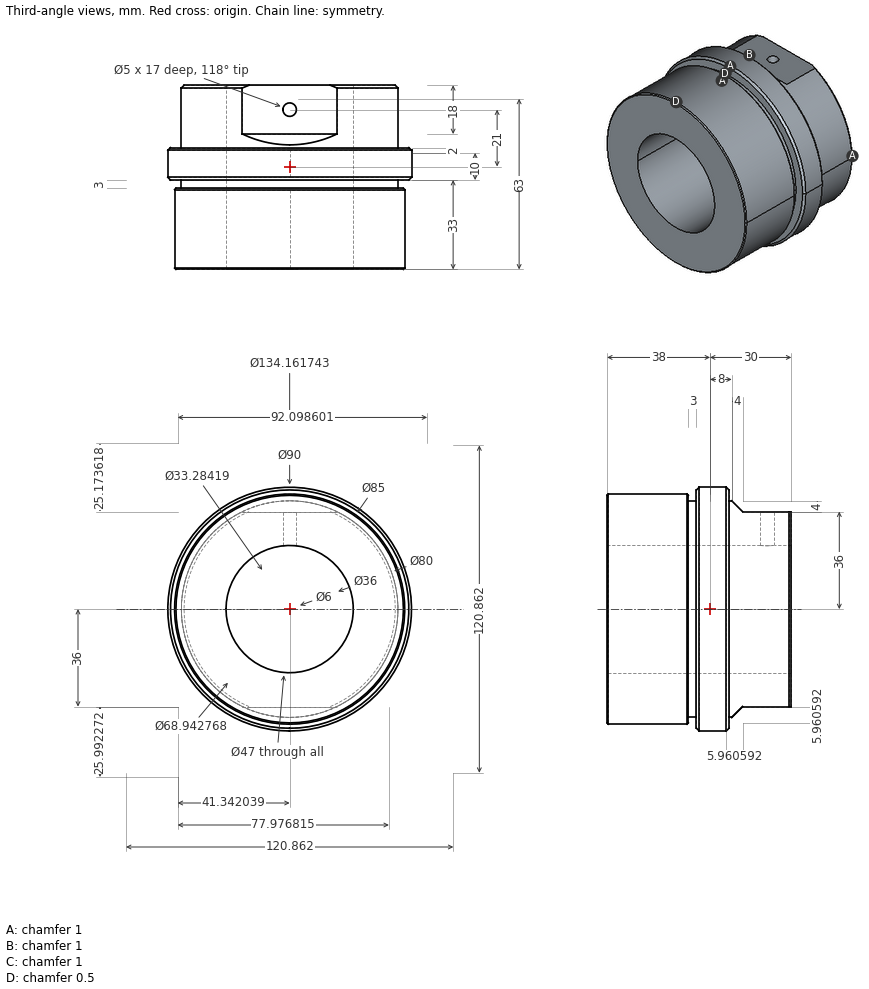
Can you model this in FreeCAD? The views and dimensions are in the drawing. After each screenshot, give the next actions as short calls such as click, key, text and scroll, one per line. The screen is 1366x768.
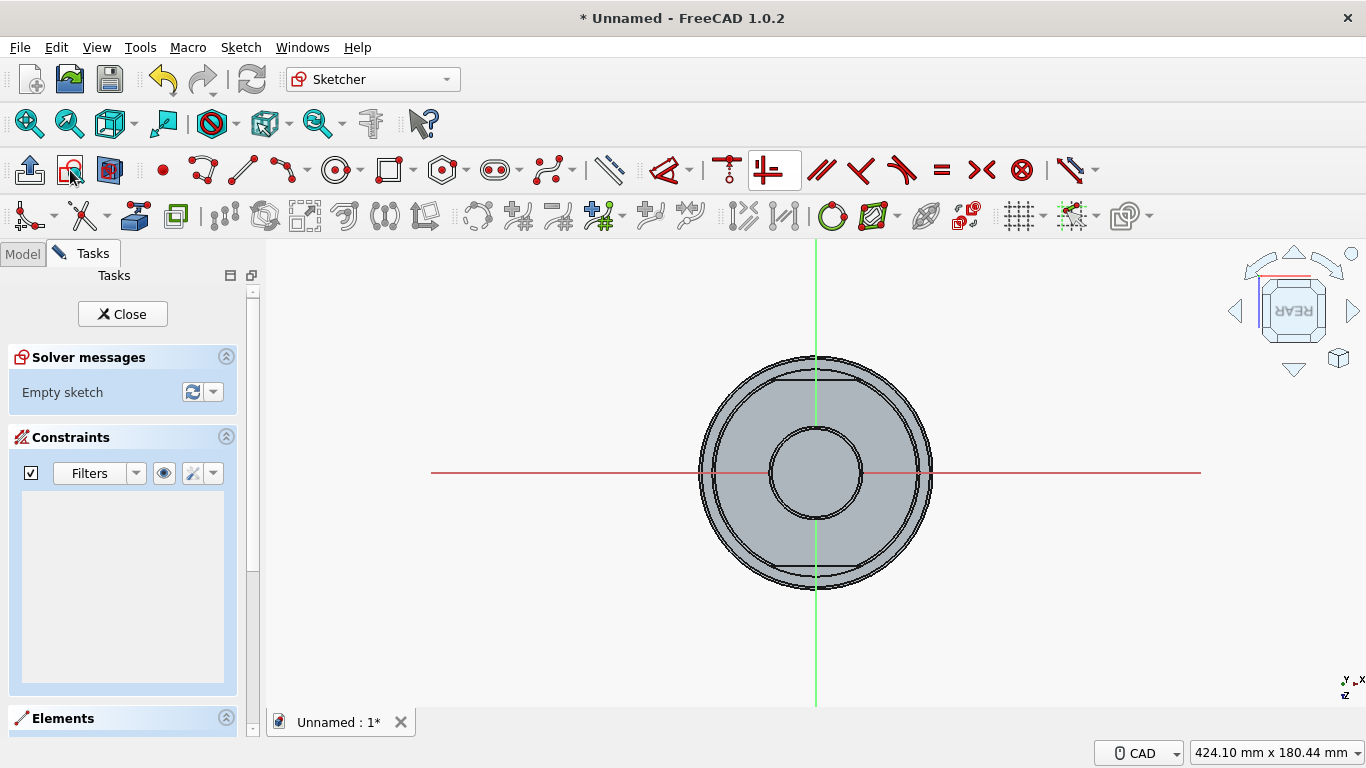
scroll(845, 473, up, 6)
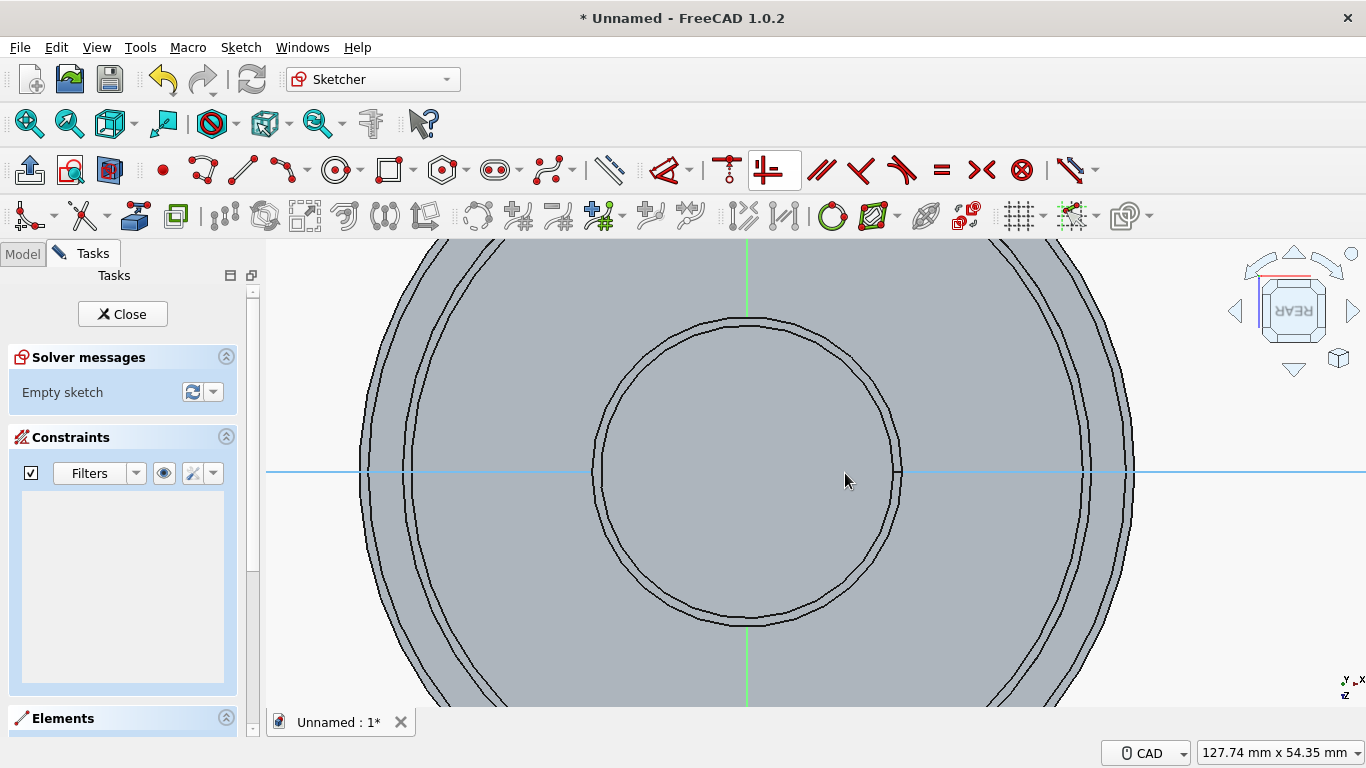
click(336, 170)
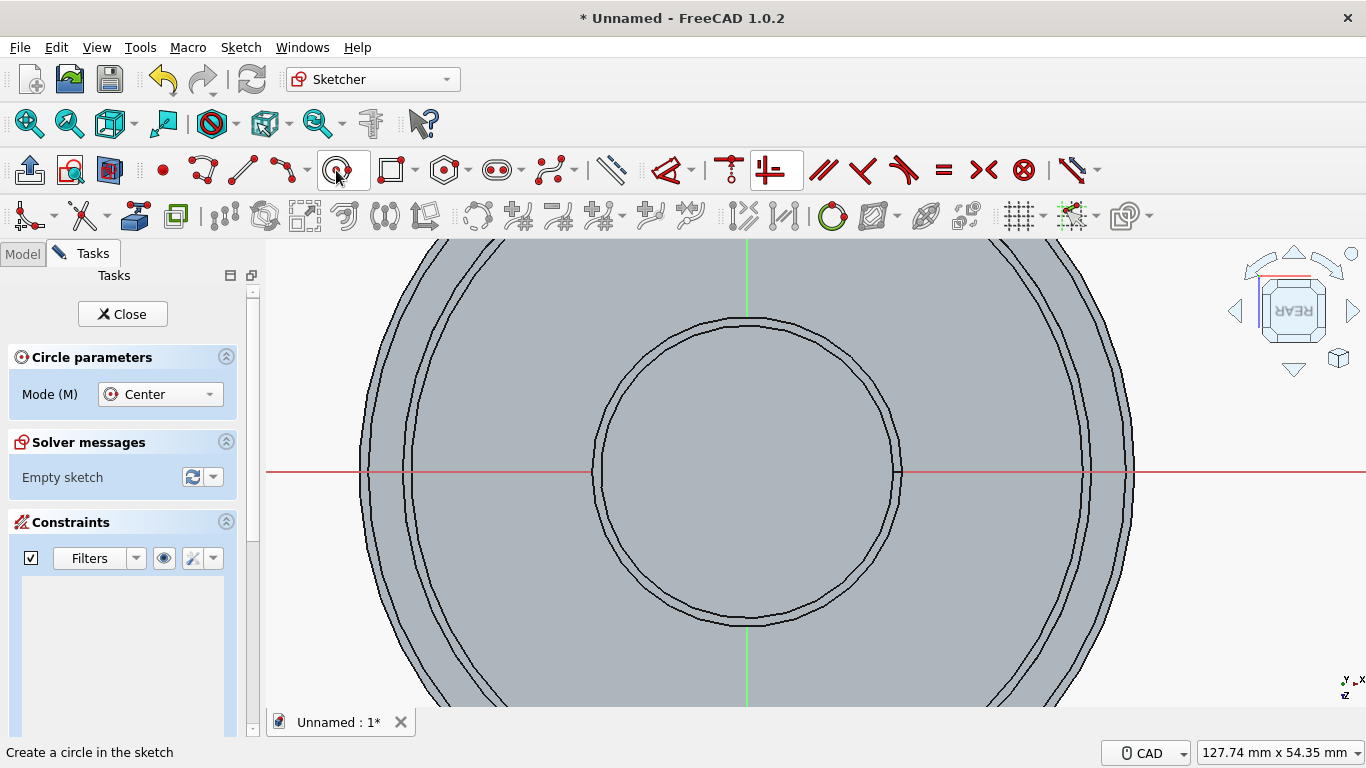
click(747, 472)
click(857, 362)
key(Escape)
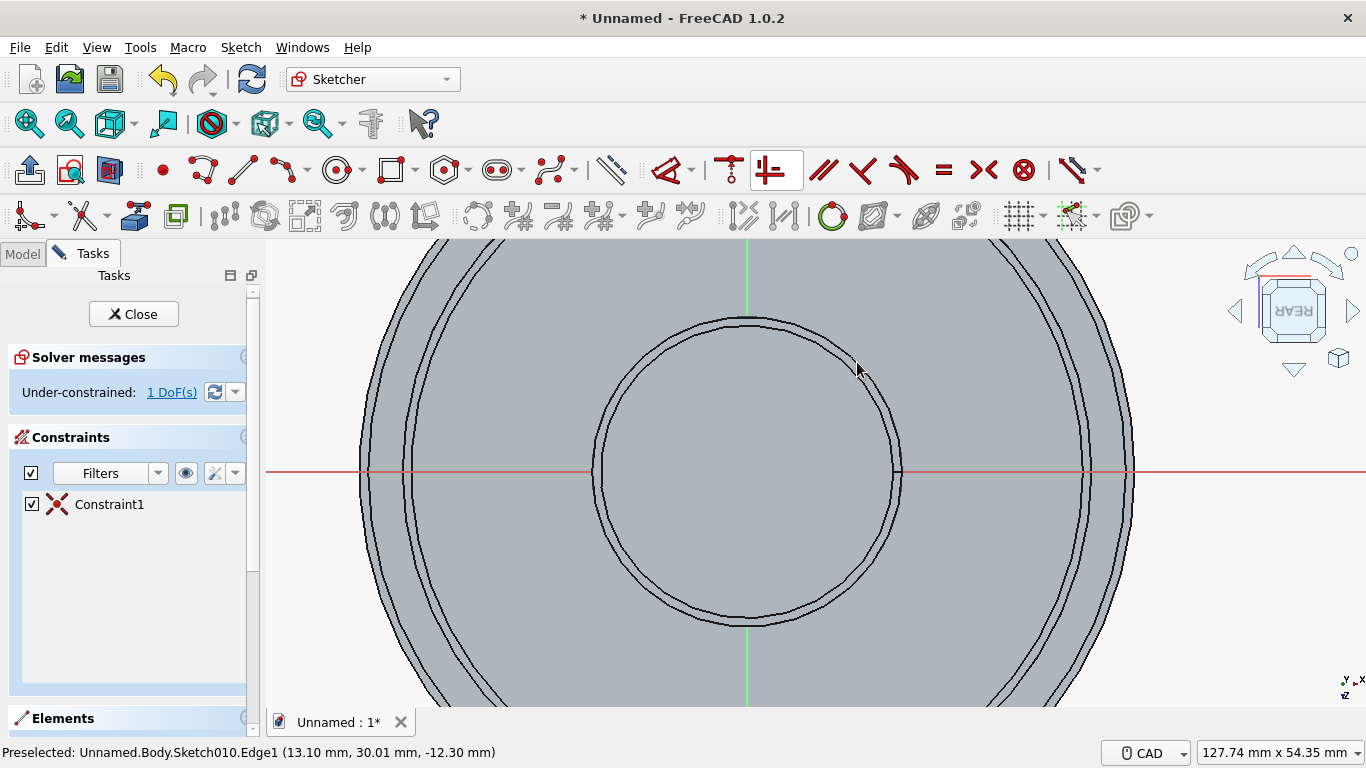
click(666, 170)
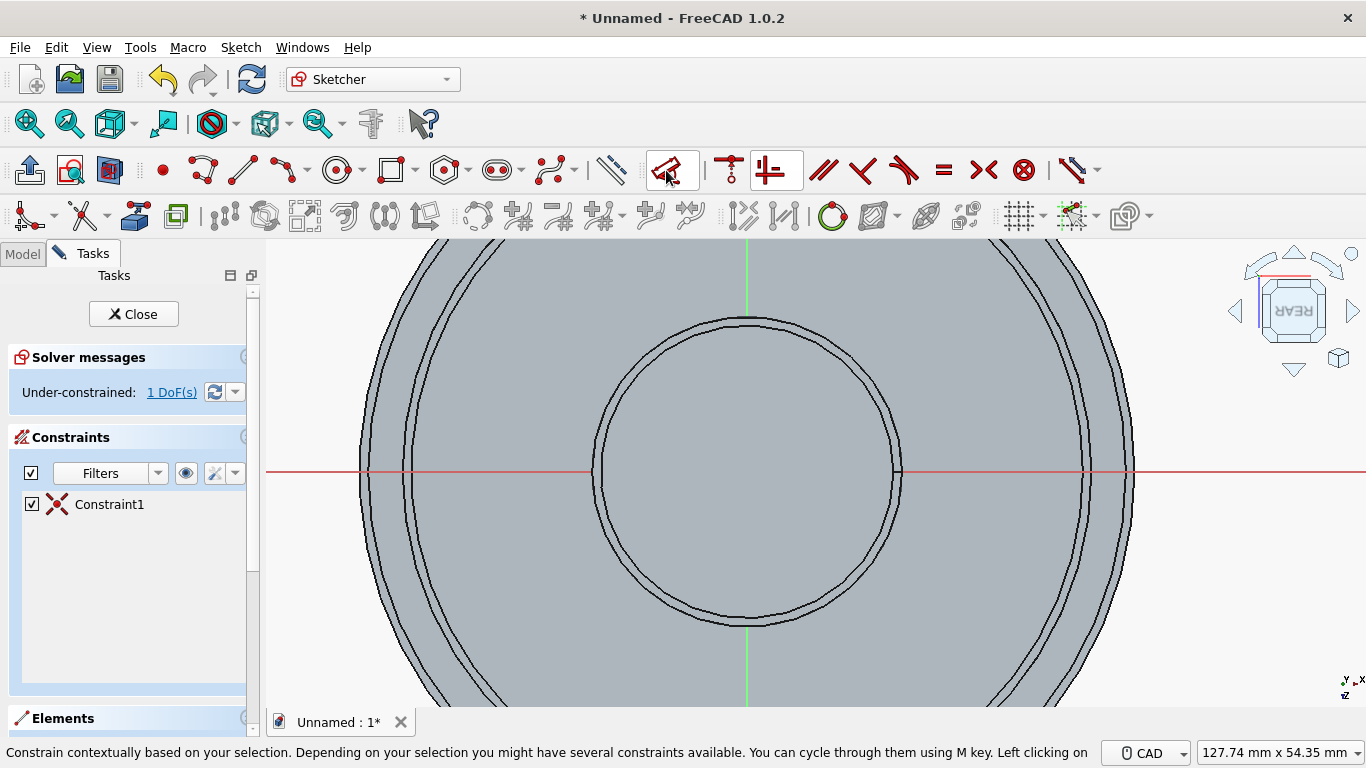
click(856, 362)
click(879, 339)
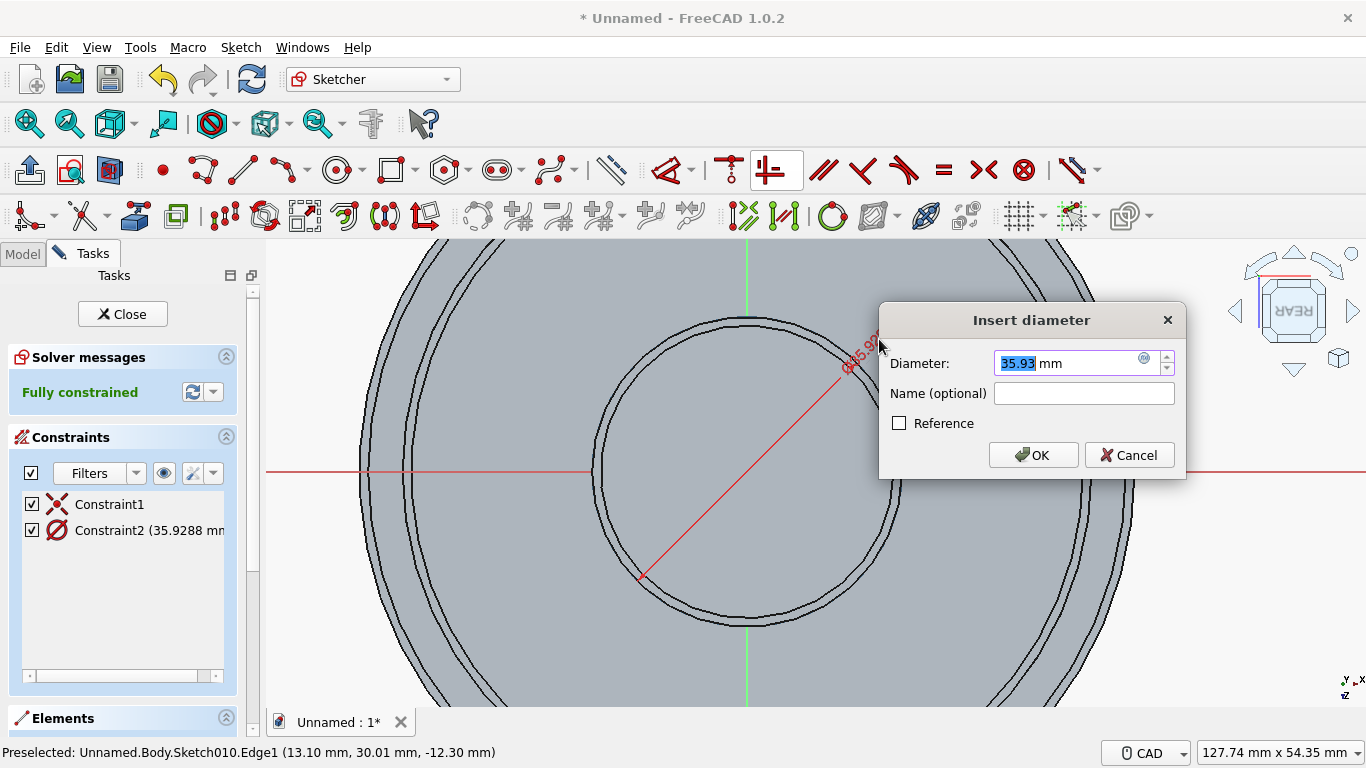
text(36)
key(Return)
key(Escape)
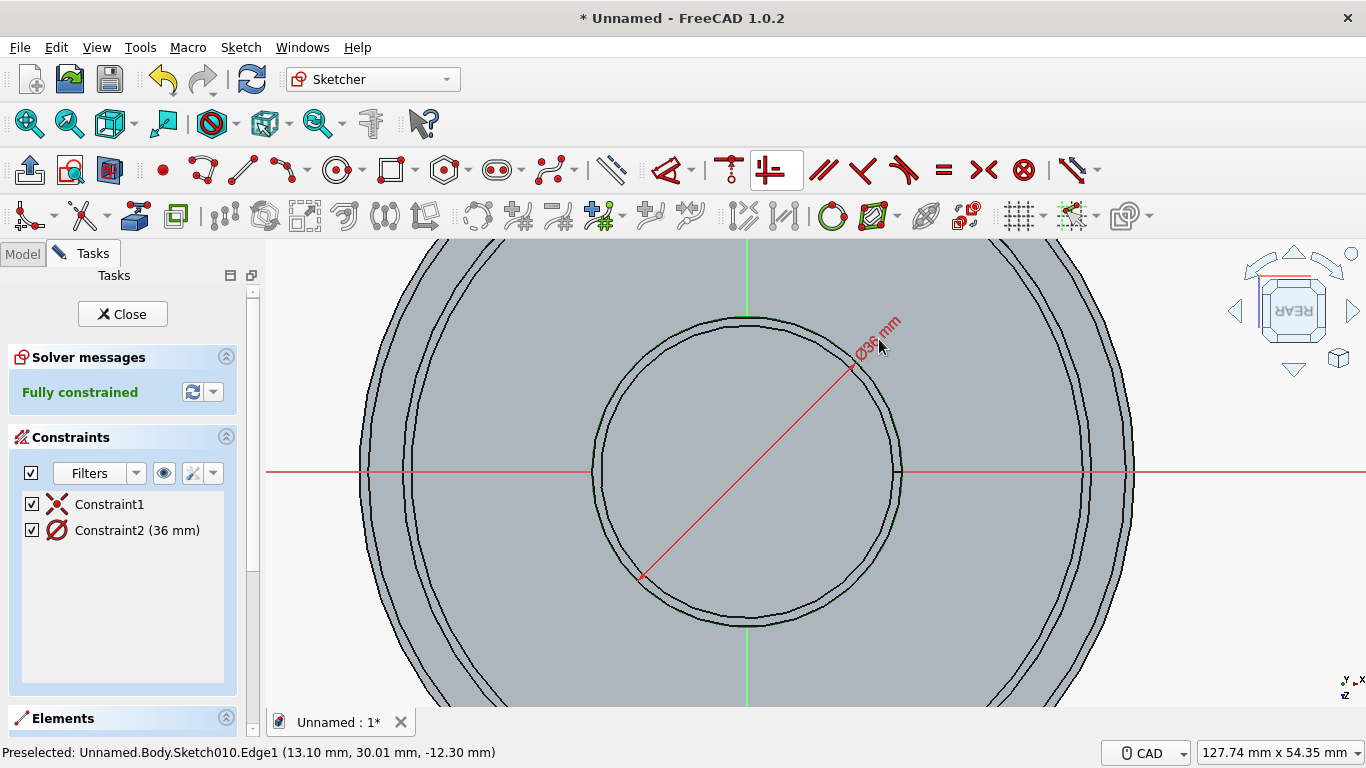
click(123, 314)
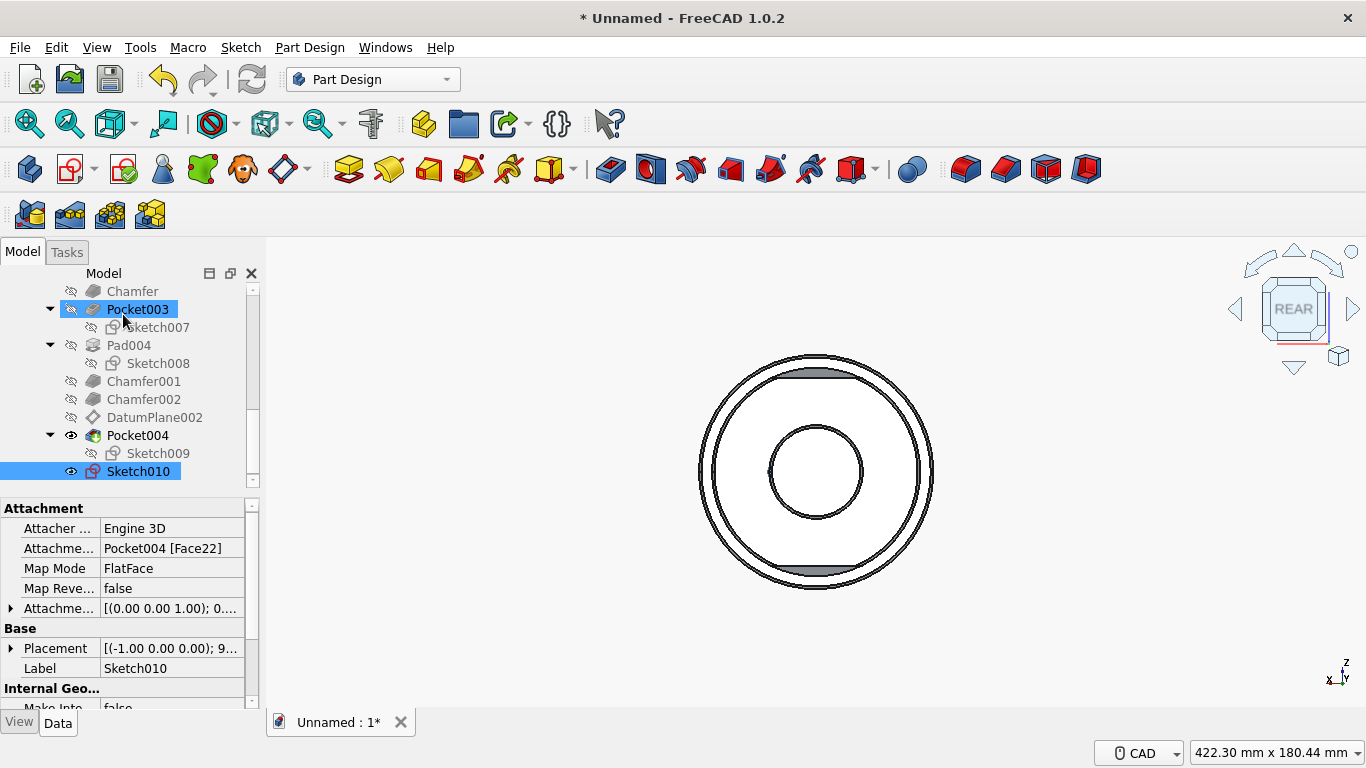
click(612, 170)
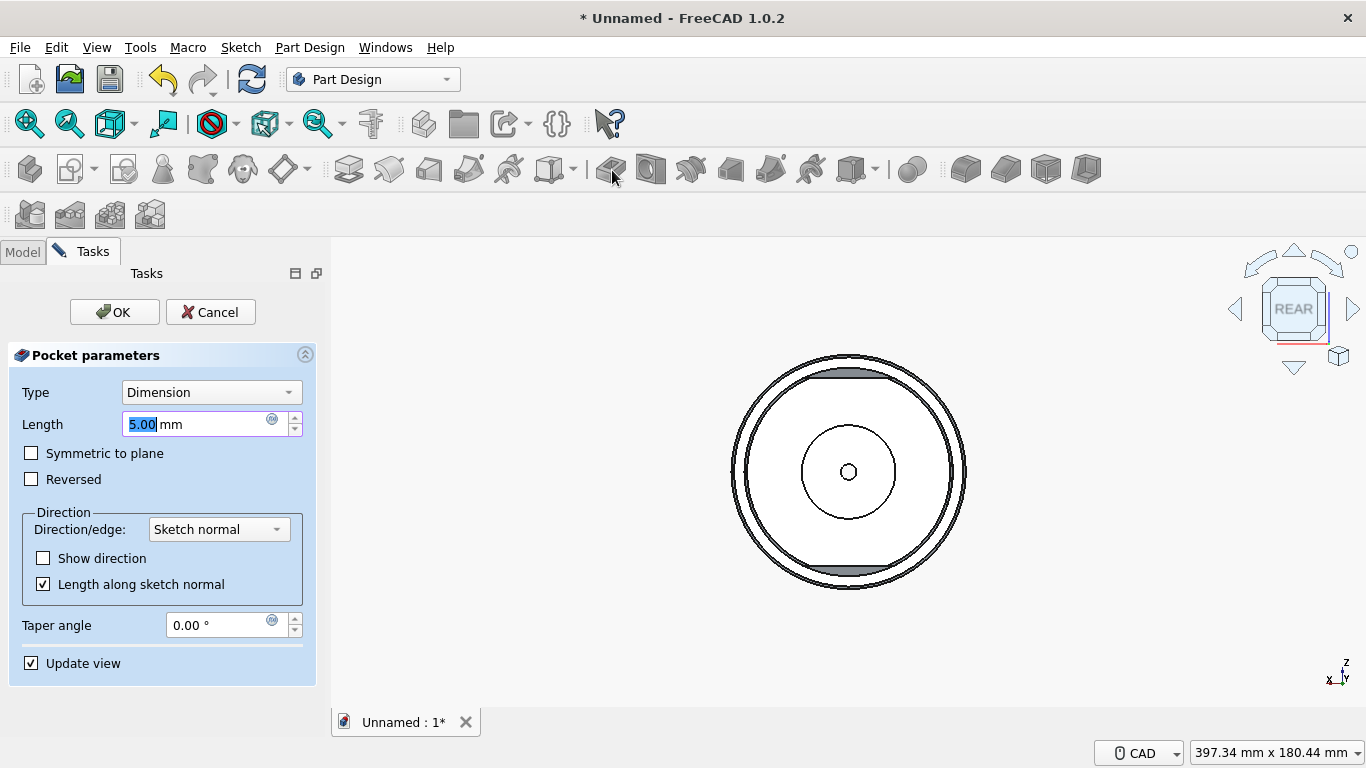
click(212, 392)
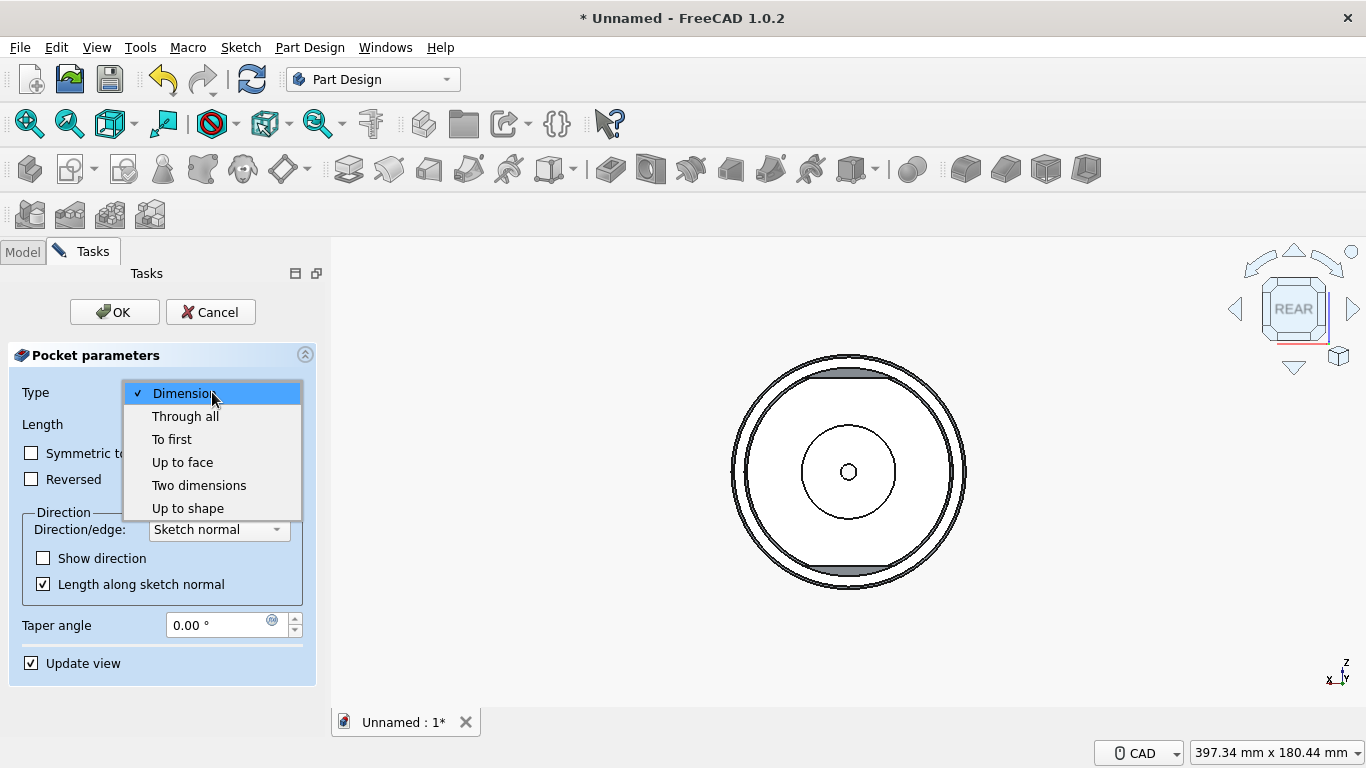
click(212, 416)